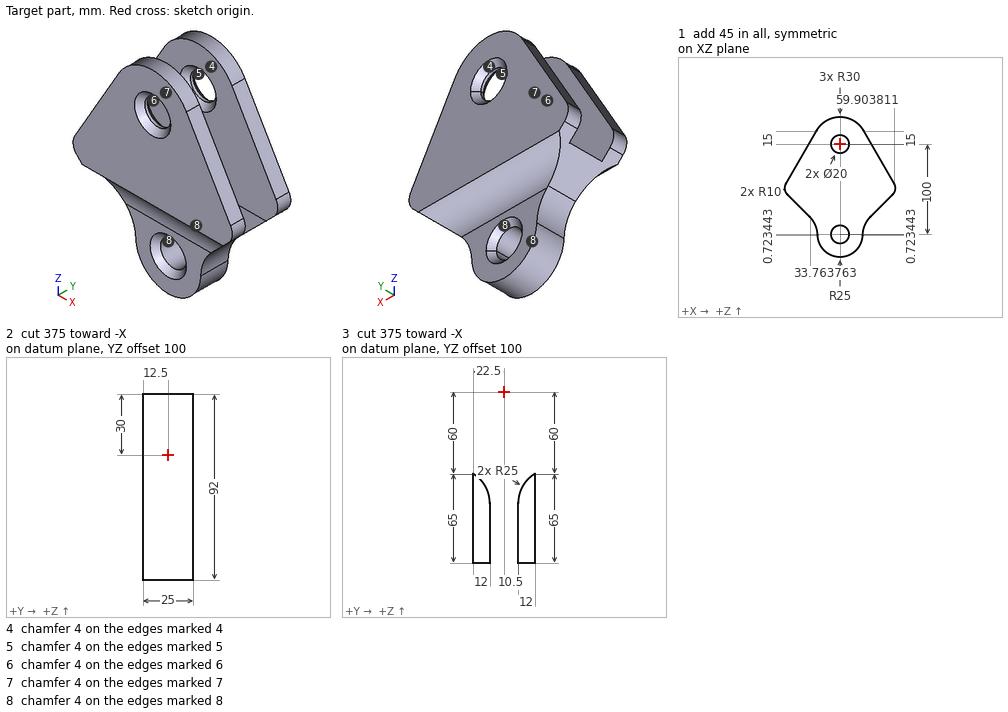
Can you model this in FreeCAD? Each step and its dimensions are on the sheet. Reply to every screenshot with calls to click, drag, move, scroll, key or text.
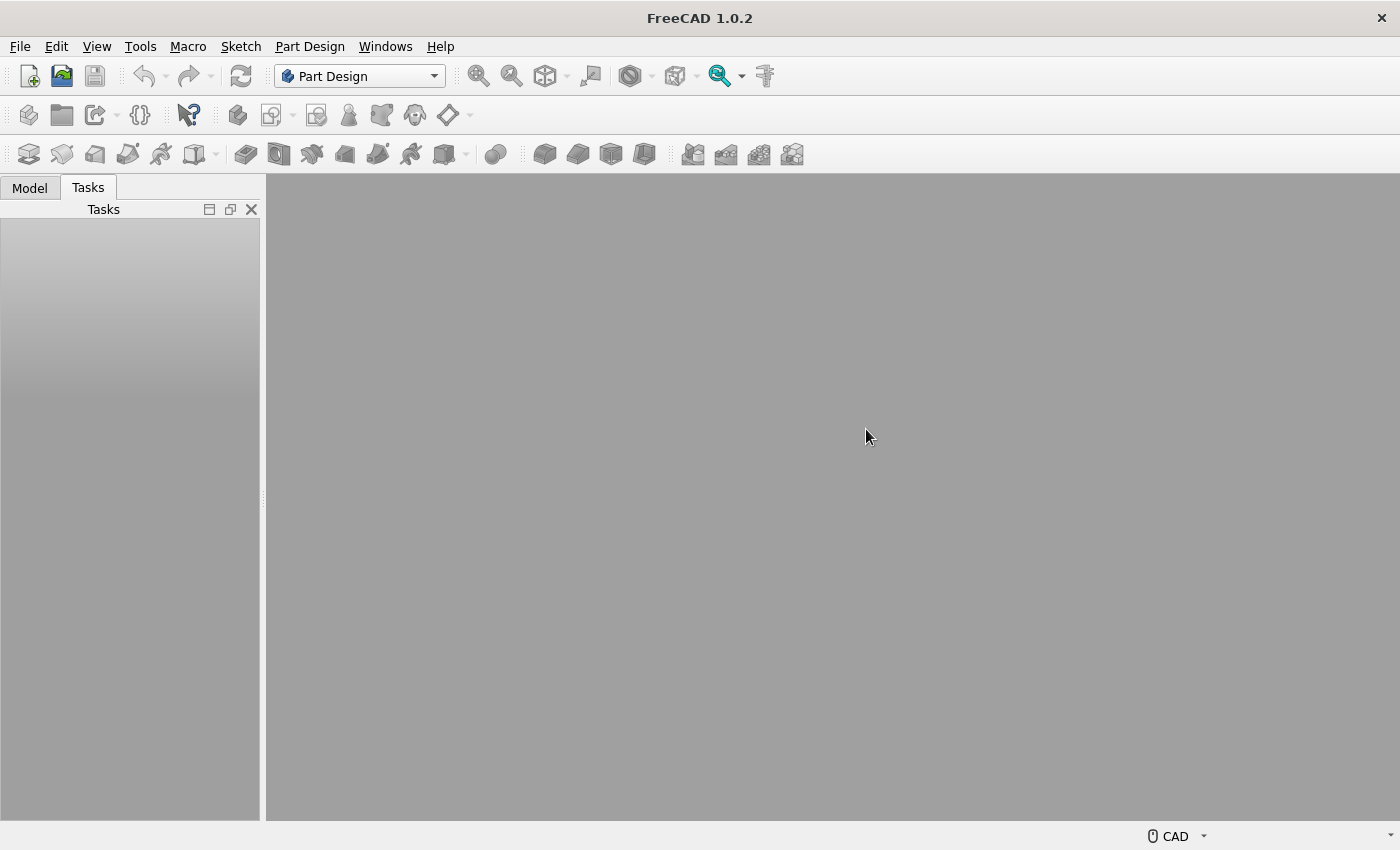
click(29, 76)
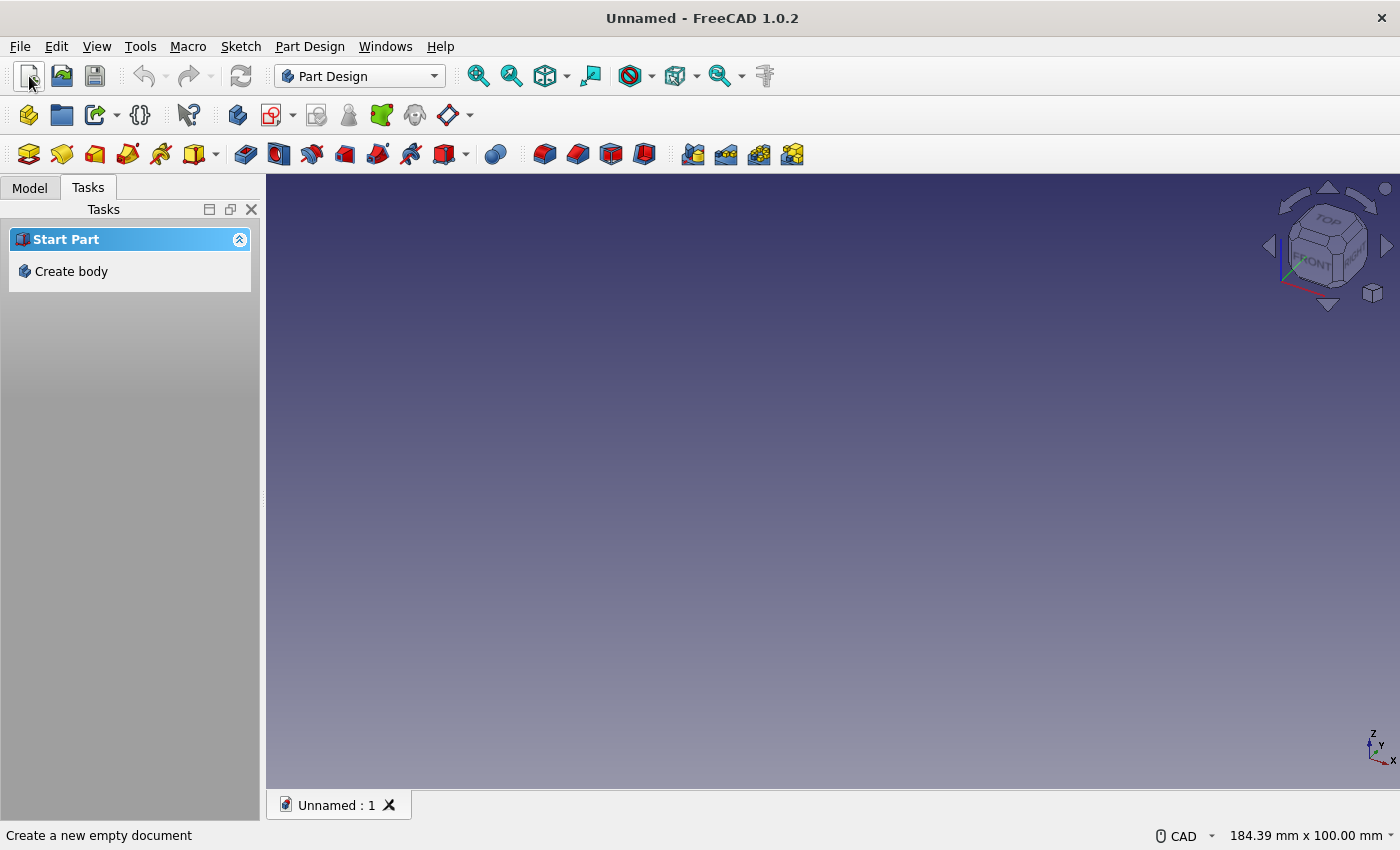
click(270, 116)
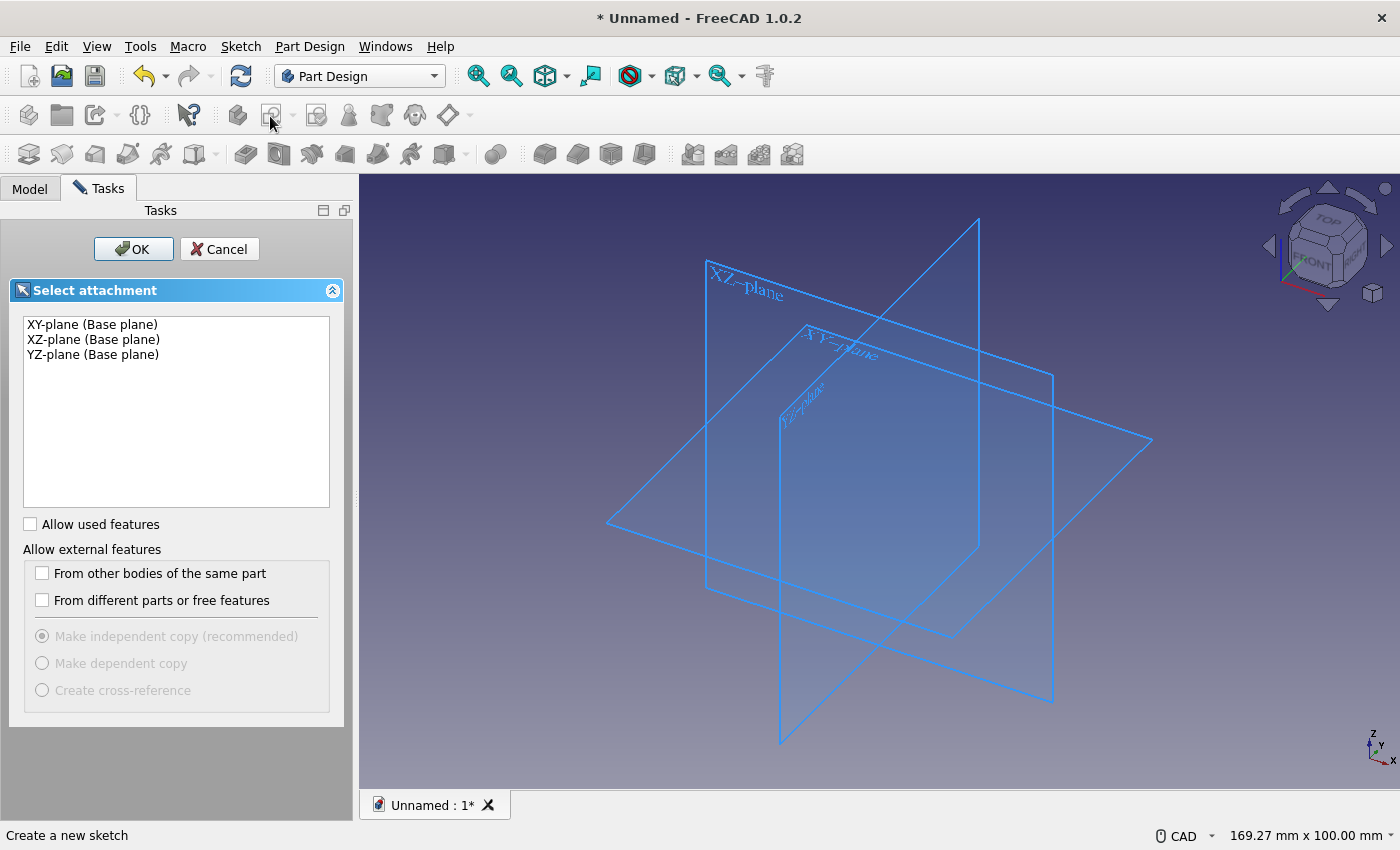
click(84, 340)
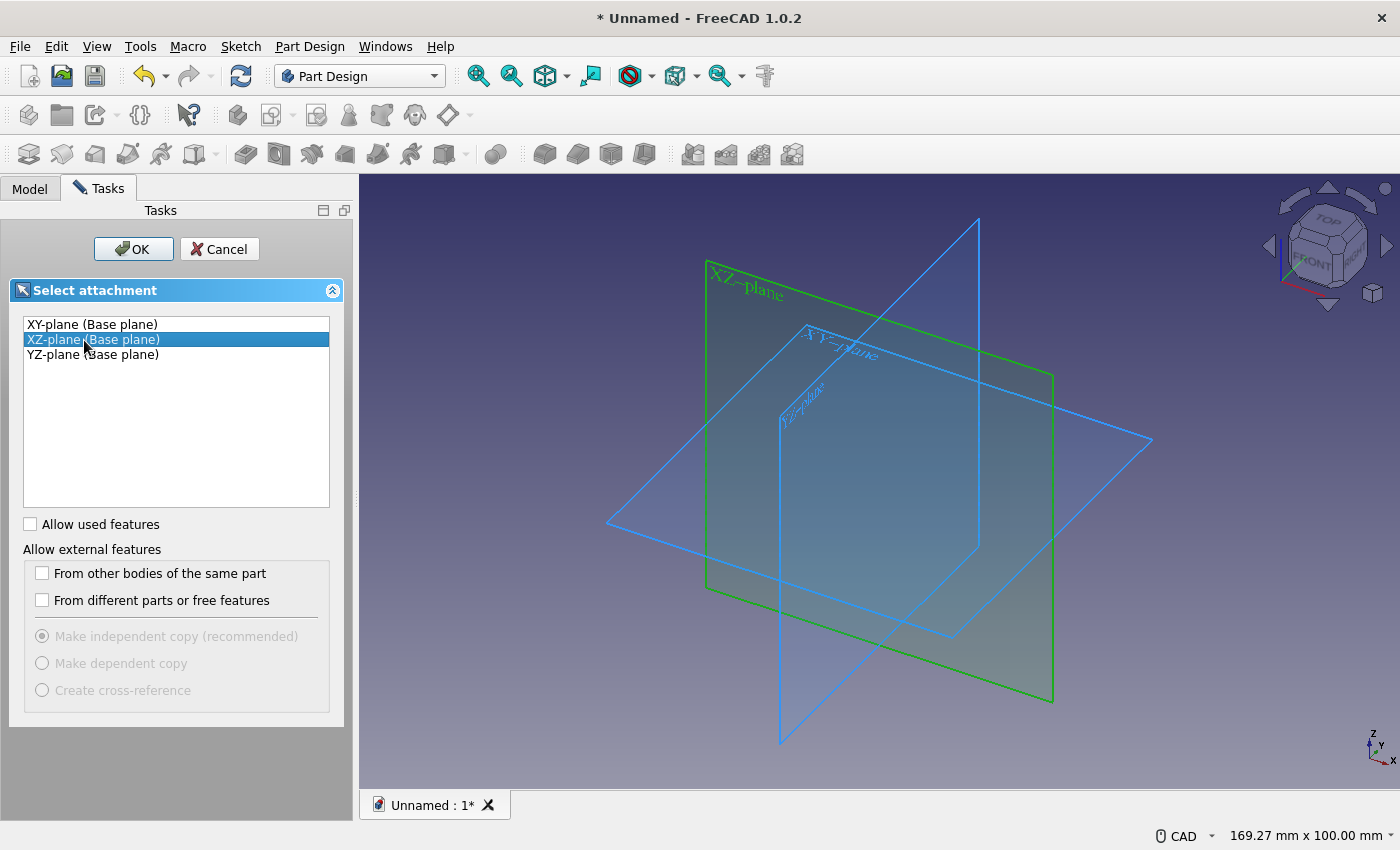
click(134, 249)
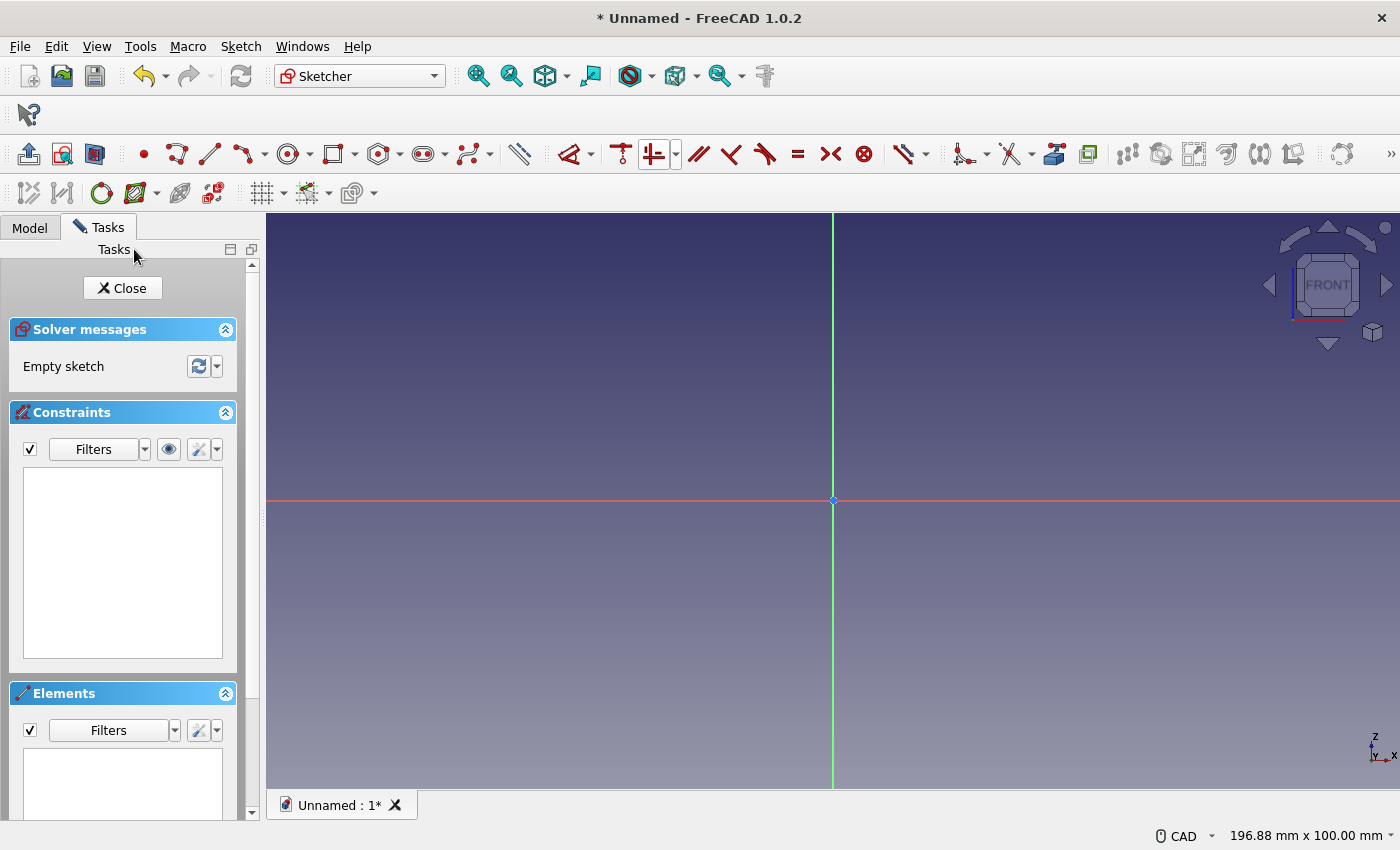
scroll(709, 278, down, 4)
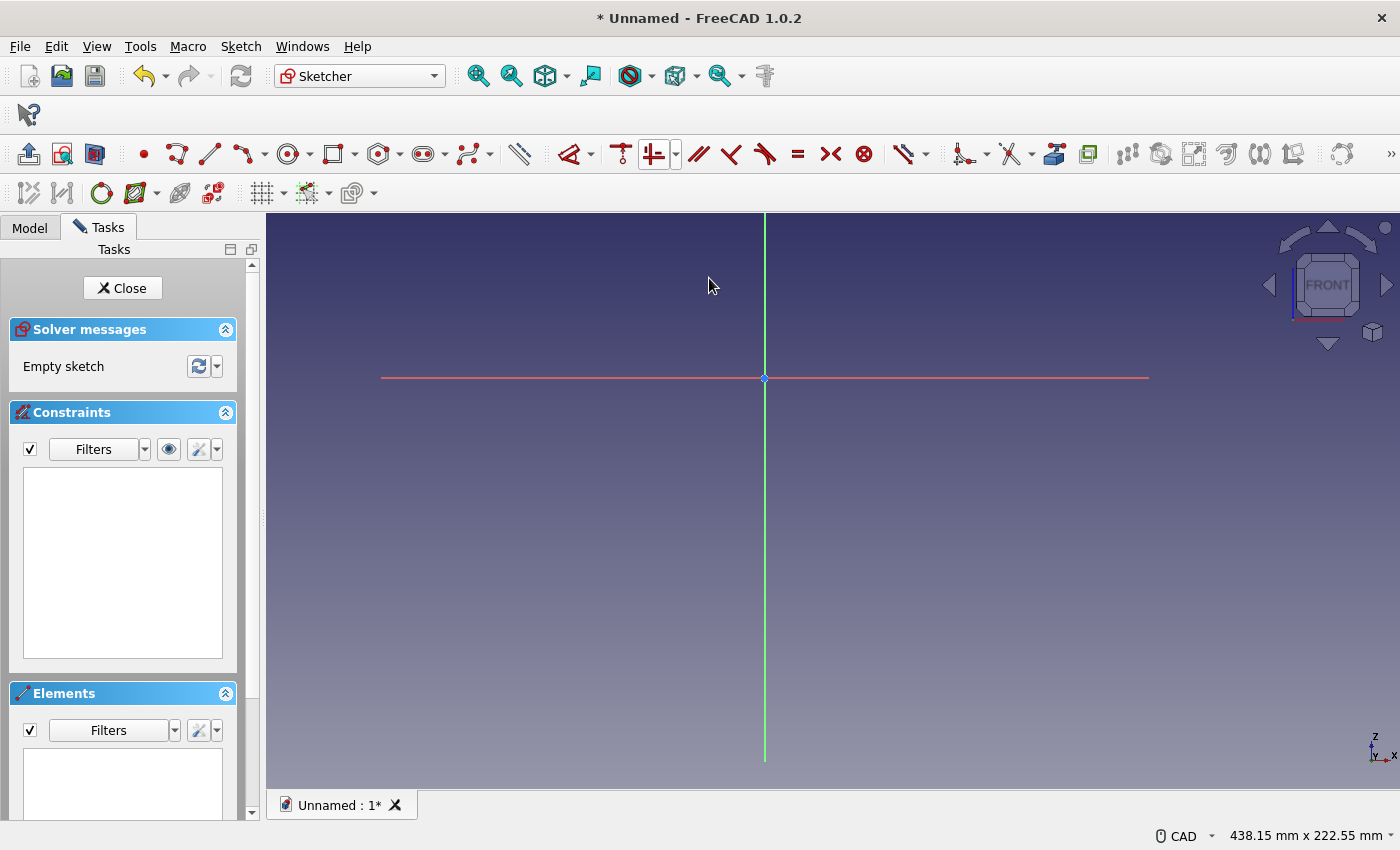
click(210, 154)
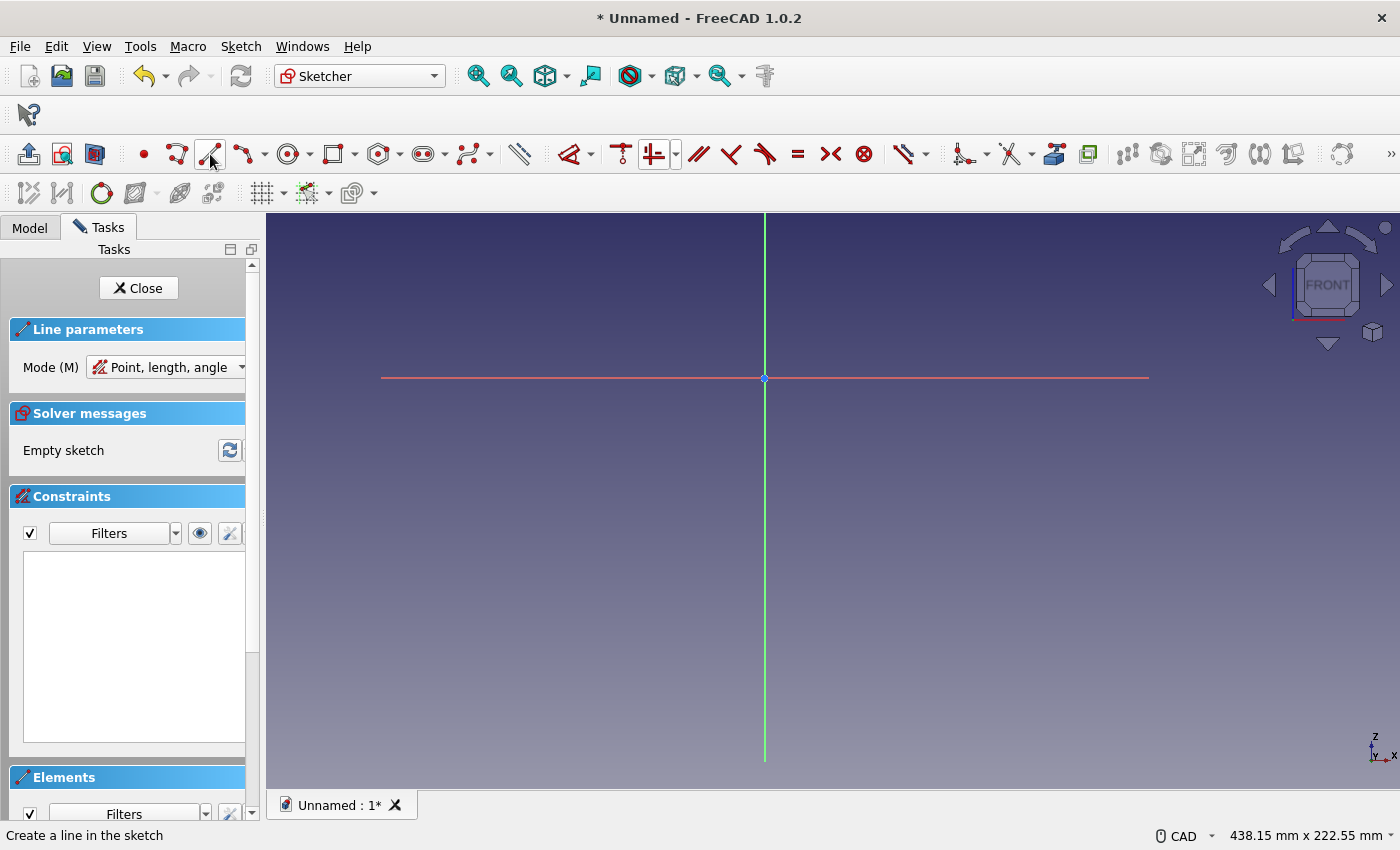
click(678, 586)
click(614, 523)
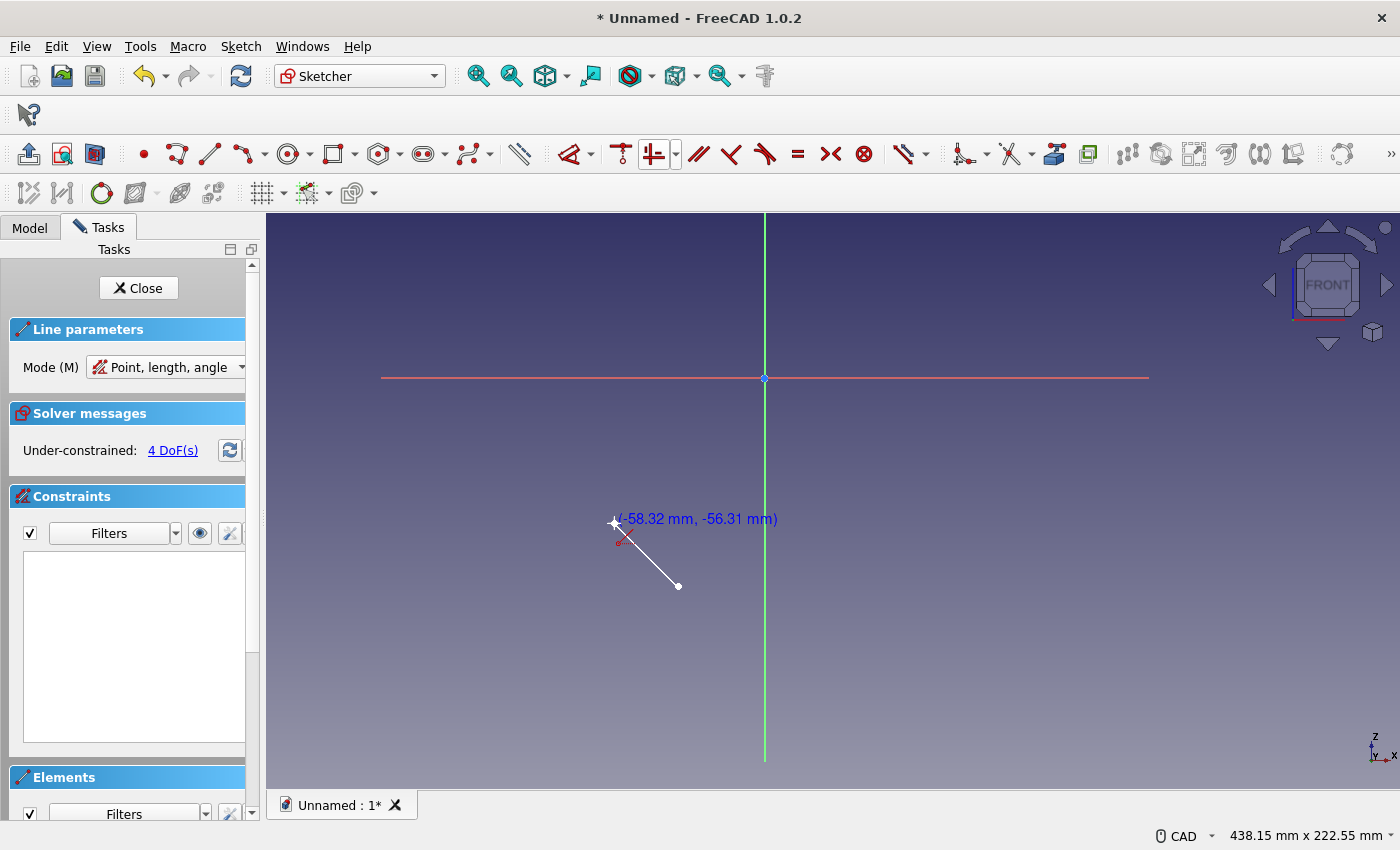
click(610, 492)
click(698, 339)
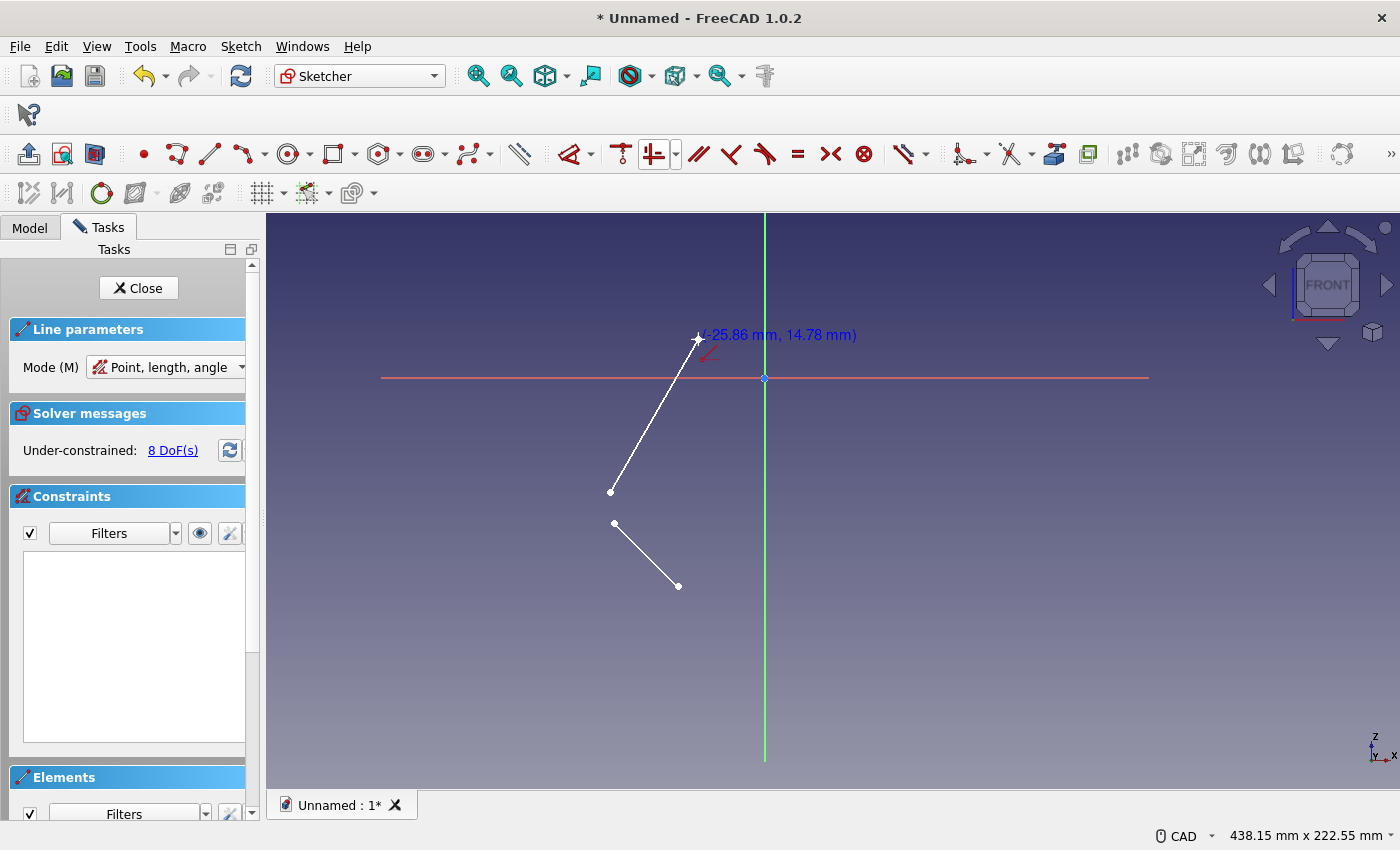
click(832, 339)
click(920, 492)